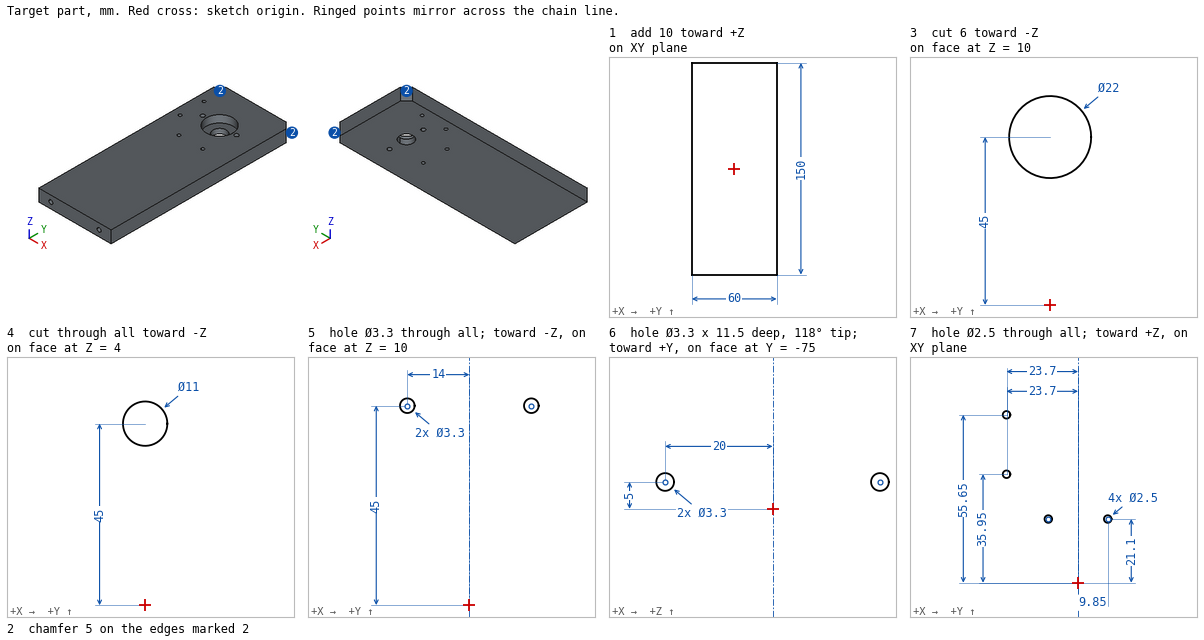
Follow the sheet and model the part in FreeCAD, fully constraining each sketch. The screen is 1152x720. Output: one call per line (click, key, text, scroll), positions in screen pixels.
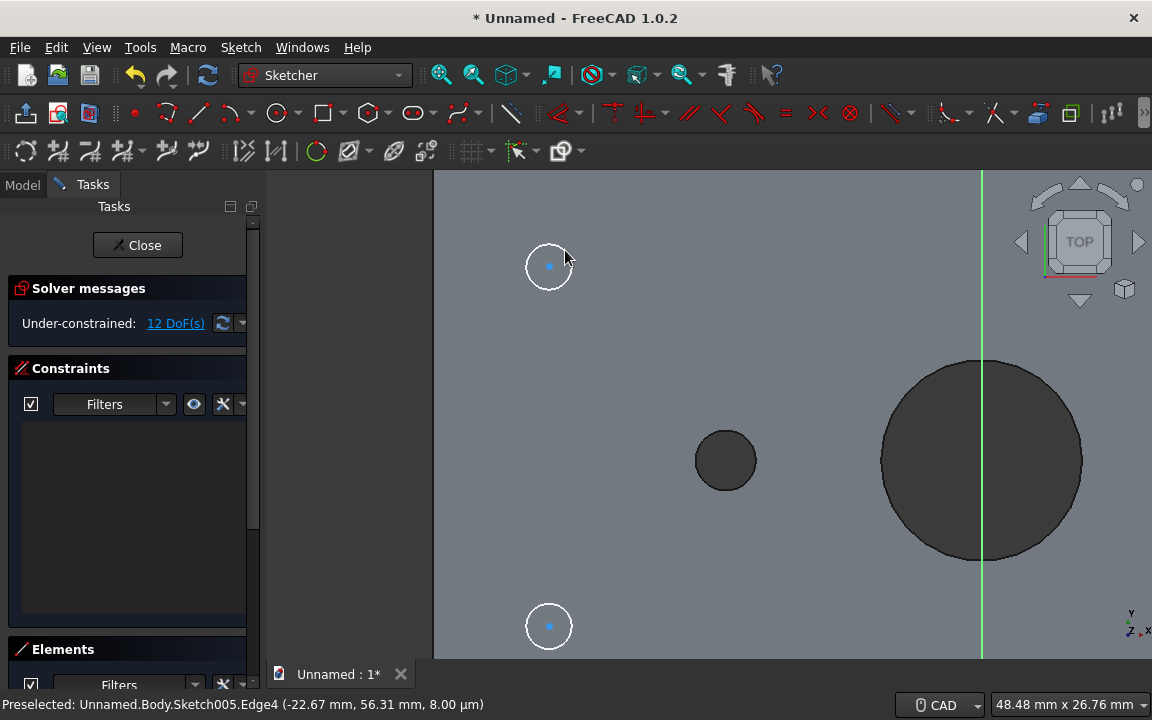
scroll(548, 264, down, 6)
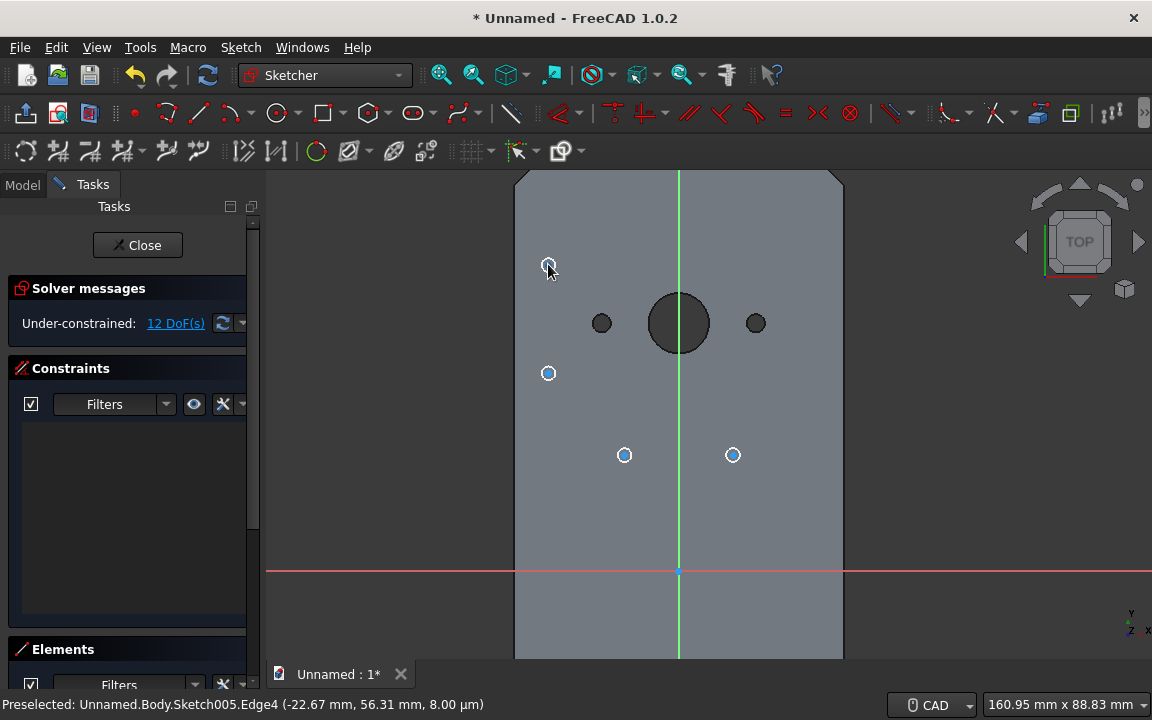
scroll(738, 450, up, 4)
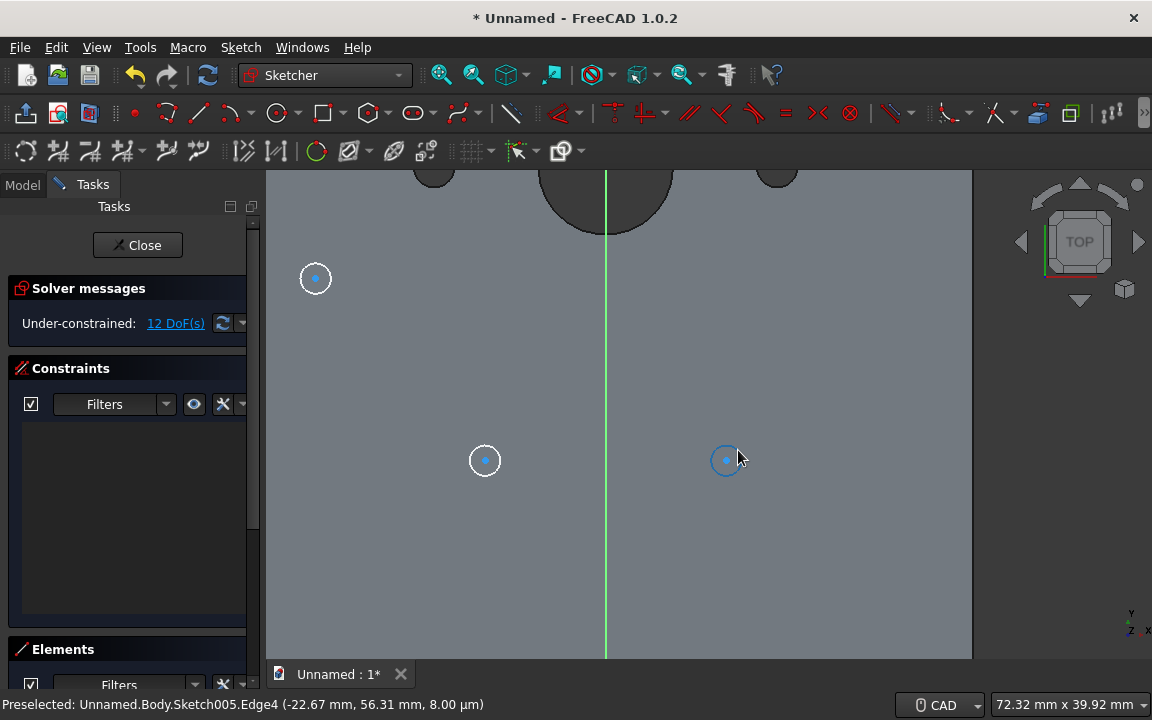
click(737, 450)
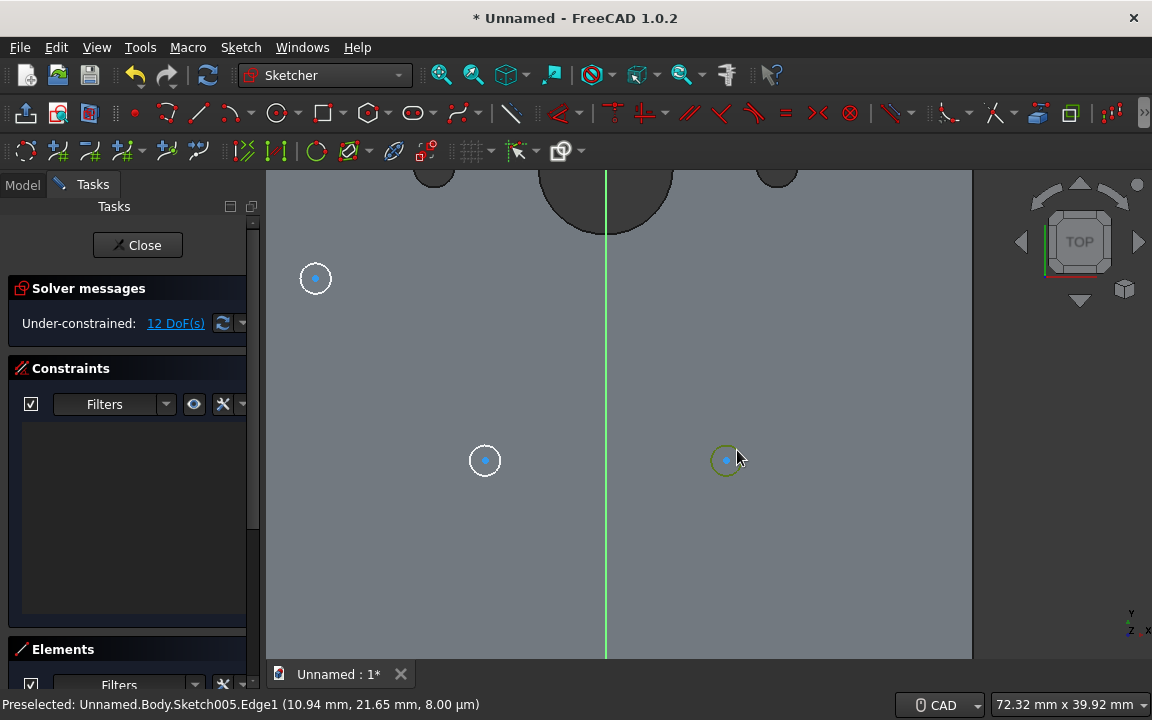
click(496, 450)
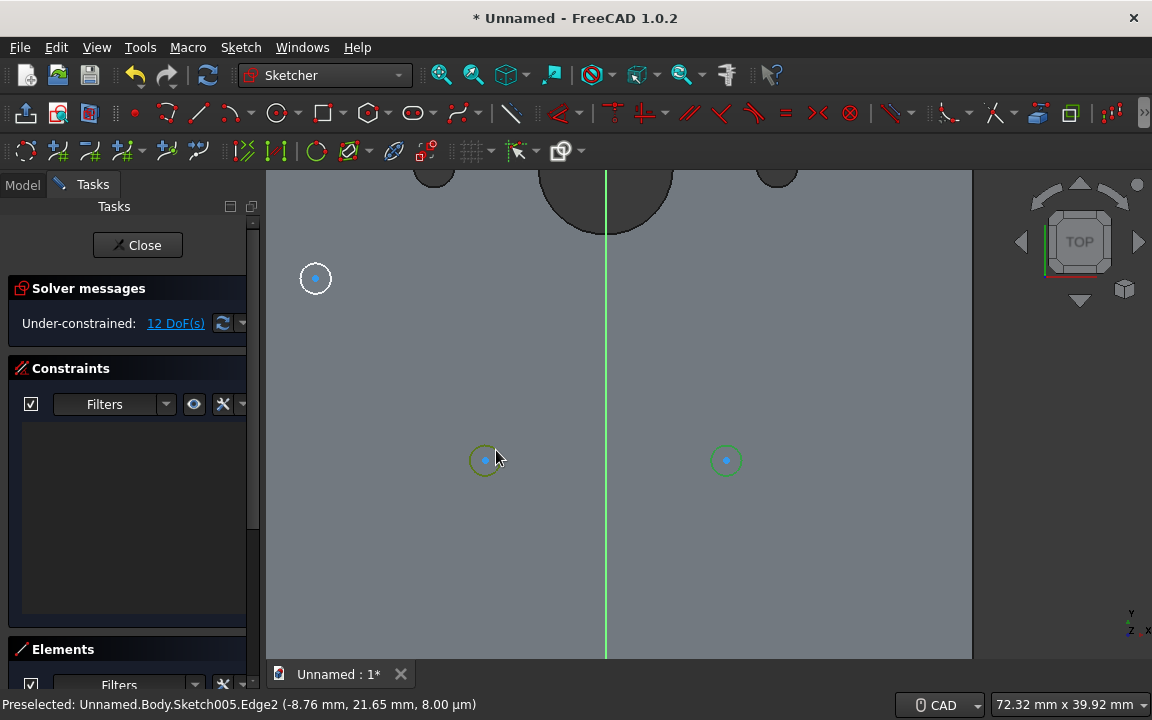
click(326, 268)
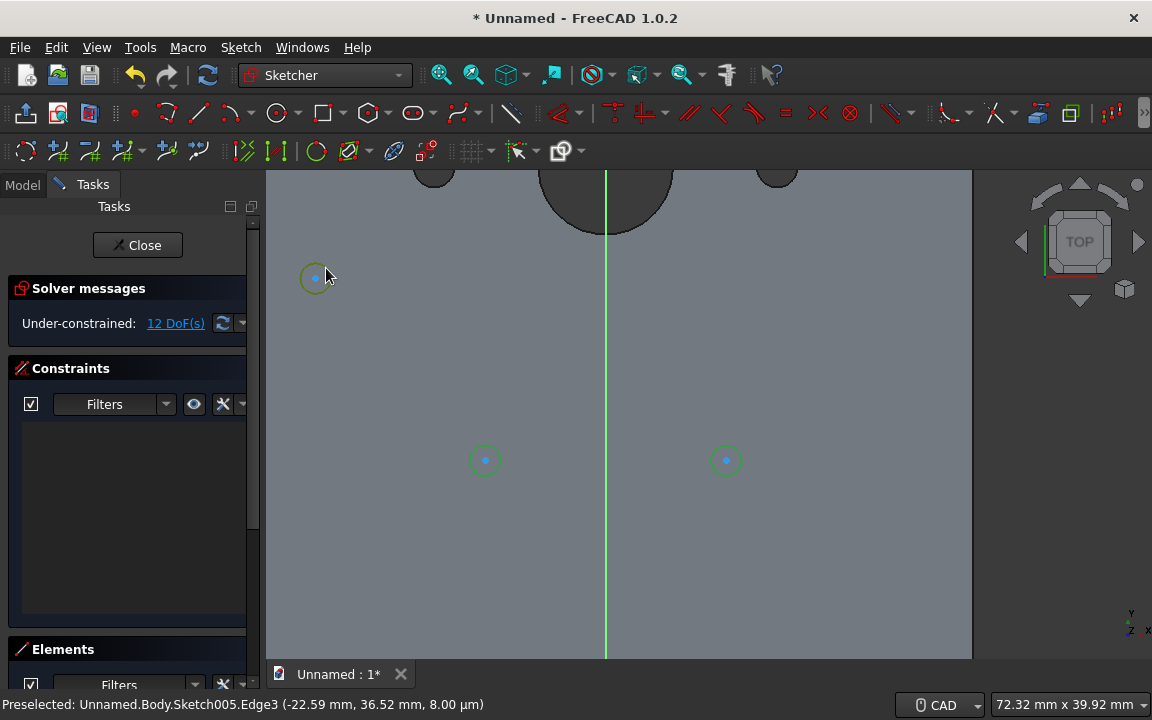
scroll(738, 451, down, 4)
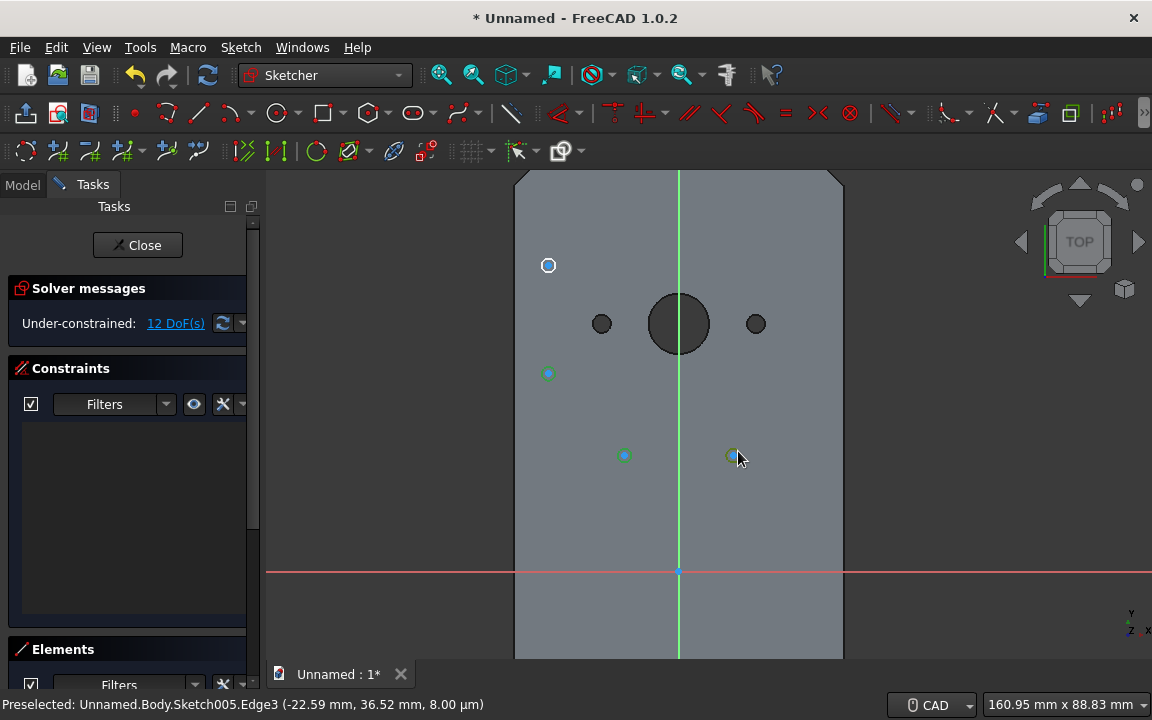
scroll(553, 261, up, 4)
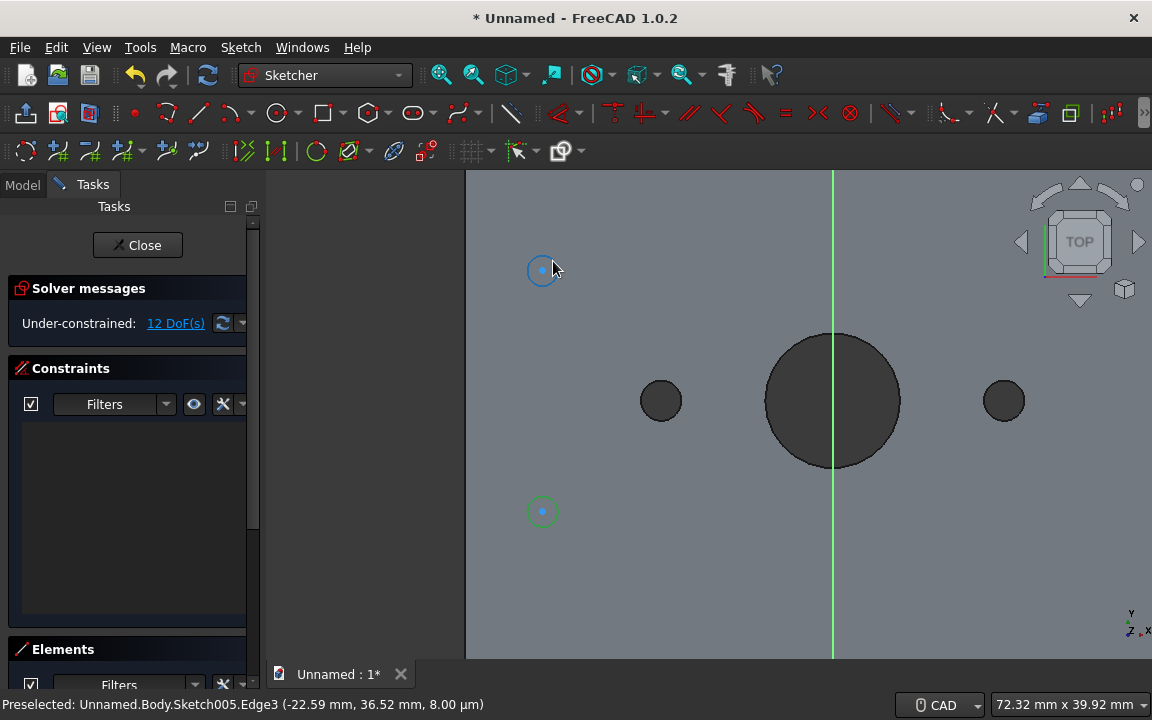
click(553, 260)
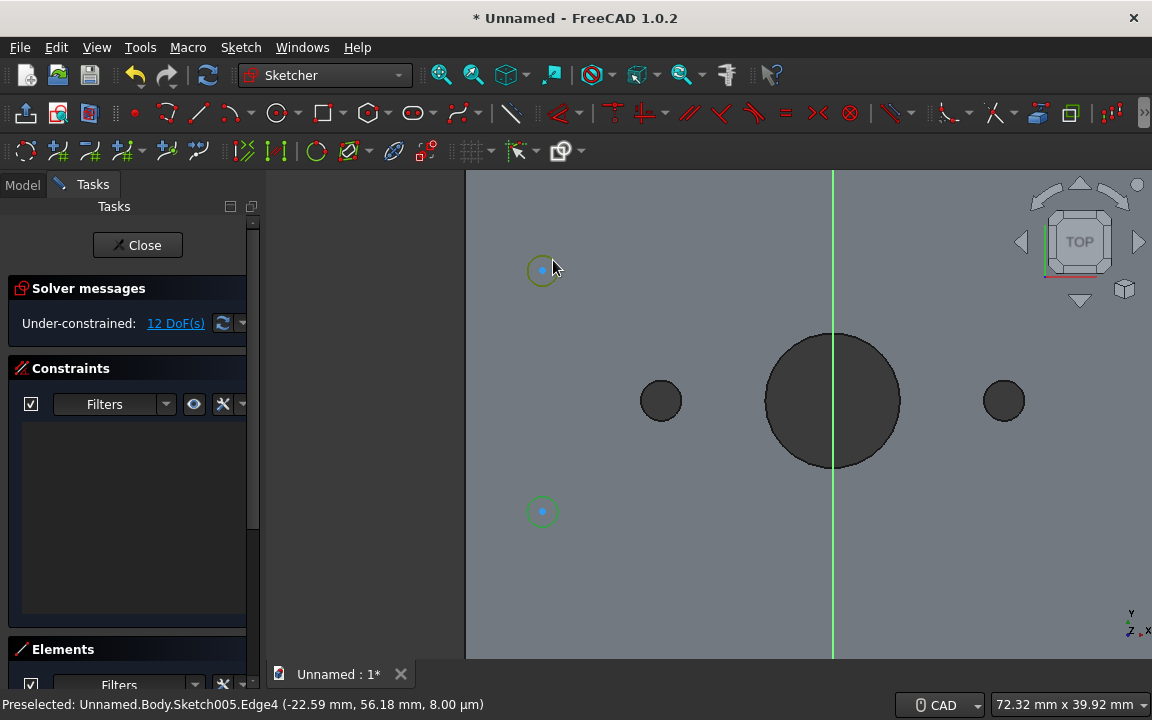
click(786, 114)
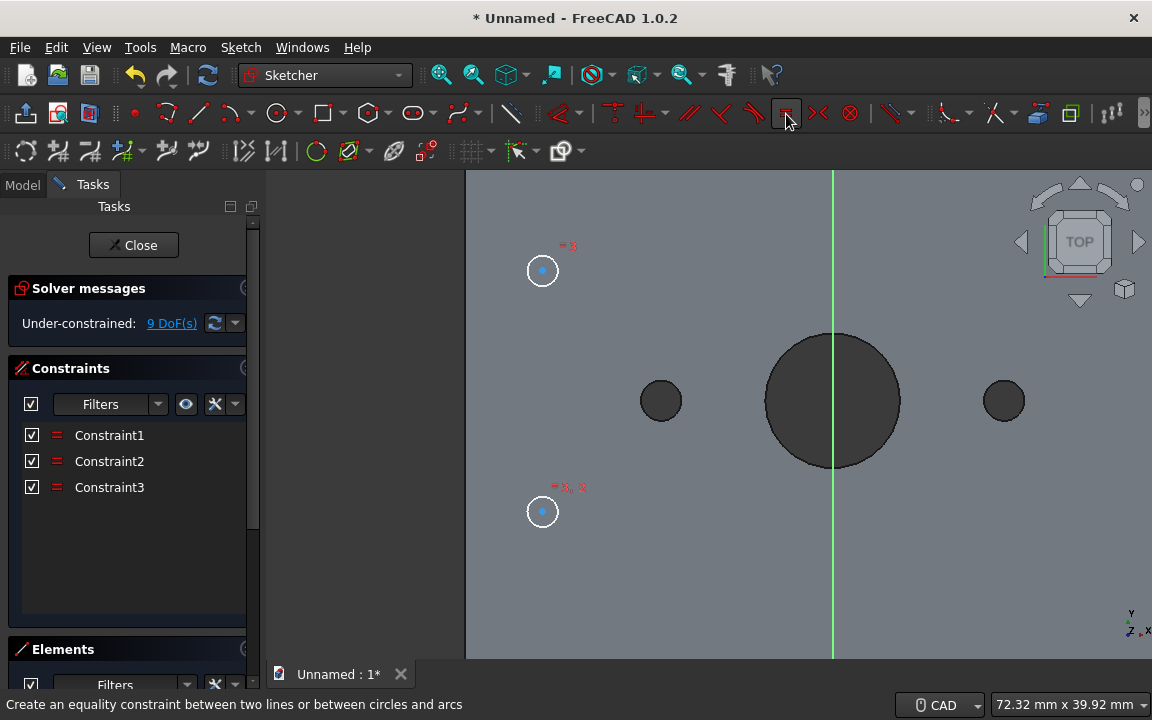
scroll(553, 260, down, 4)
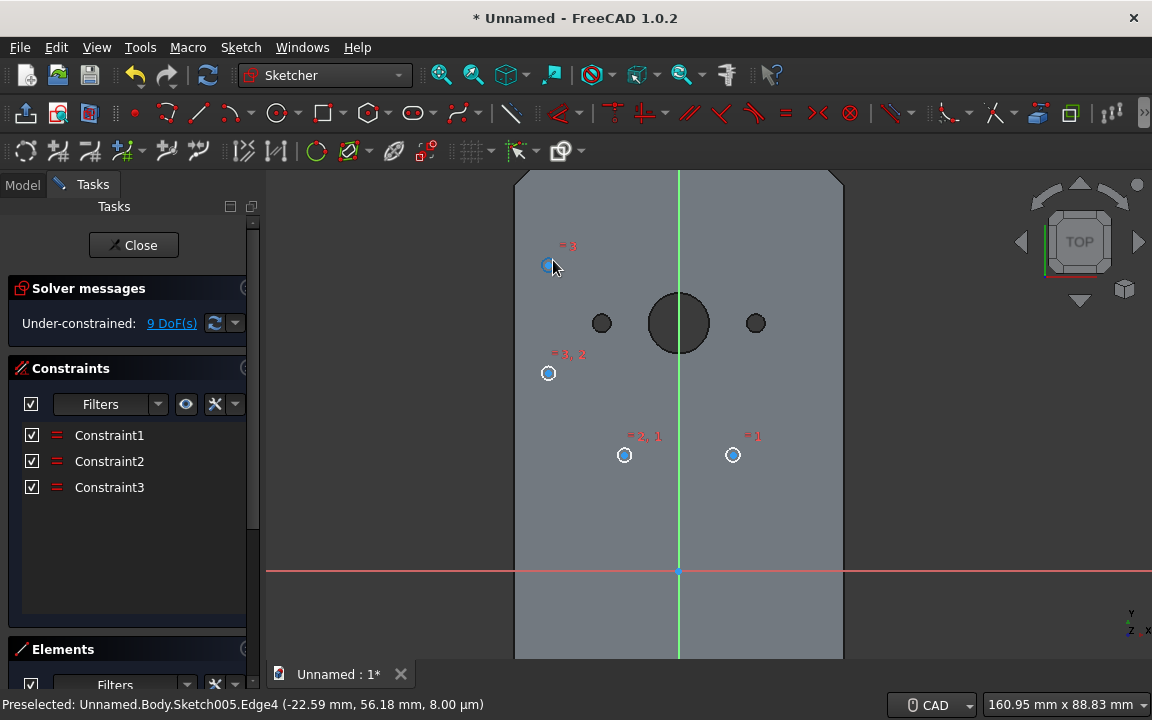
click(733, 455)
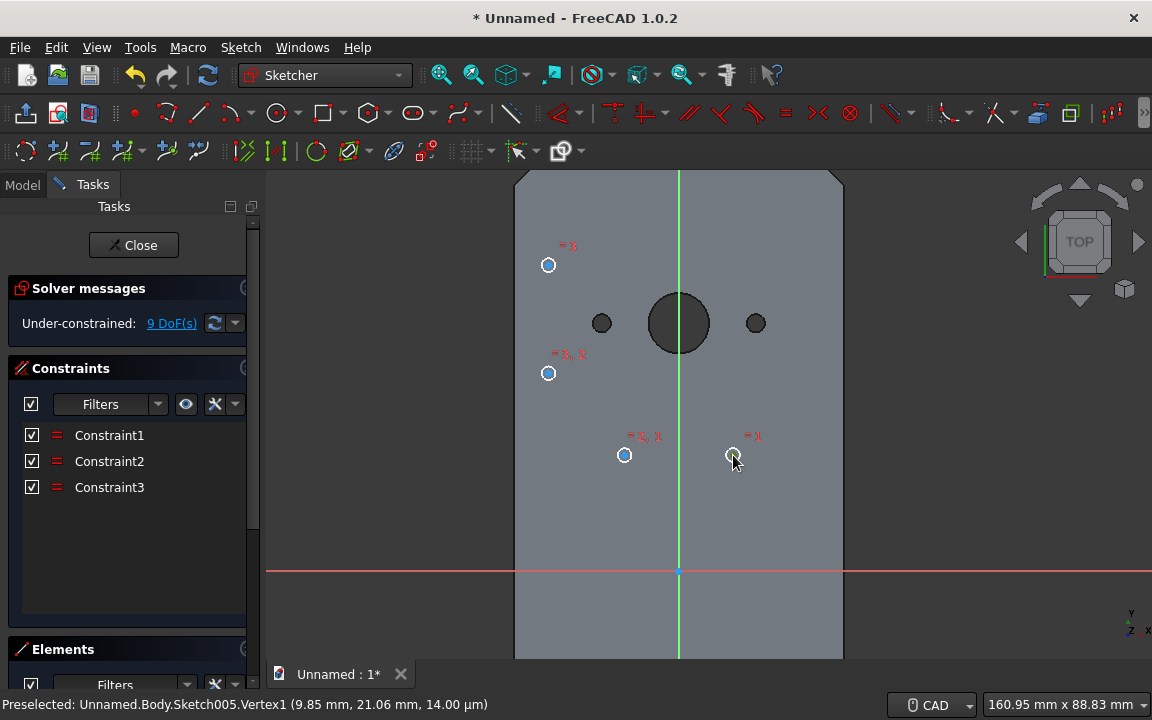
click(625, 455)